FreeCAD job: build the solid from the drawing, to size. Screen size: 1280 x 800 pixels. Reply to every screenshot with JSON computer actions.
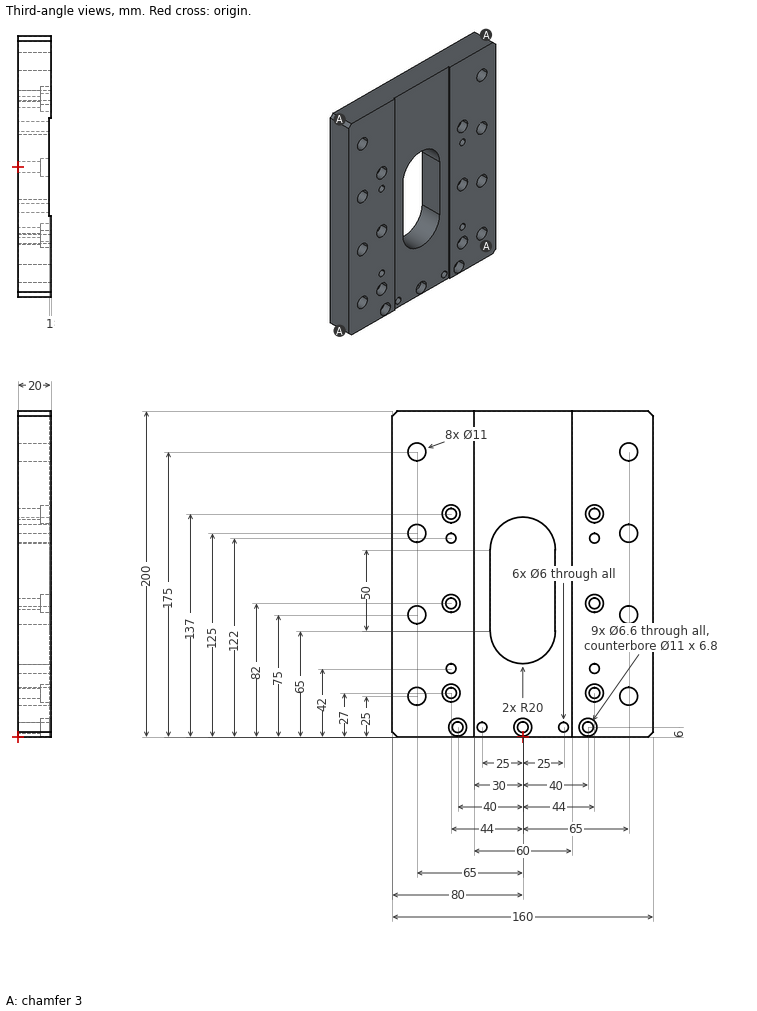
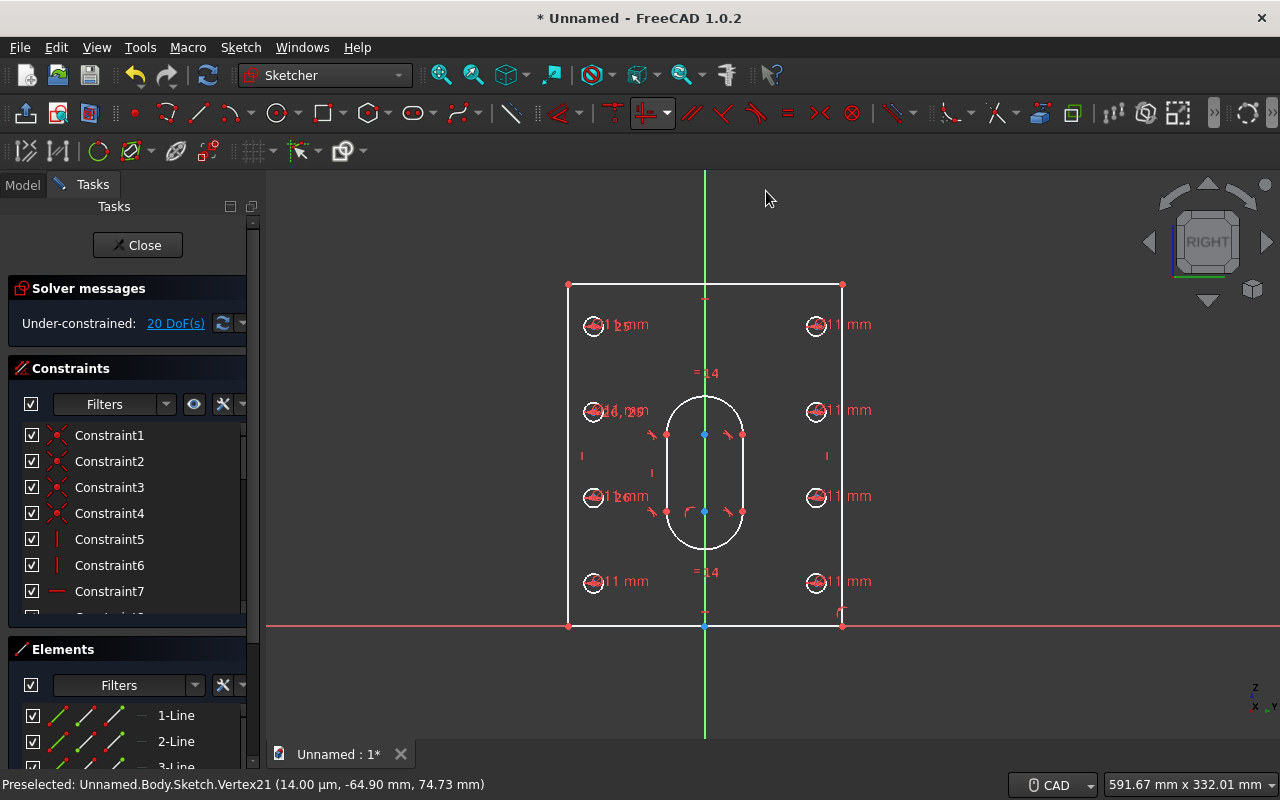
{"action": "left_click", "coordinate": [594, 498]}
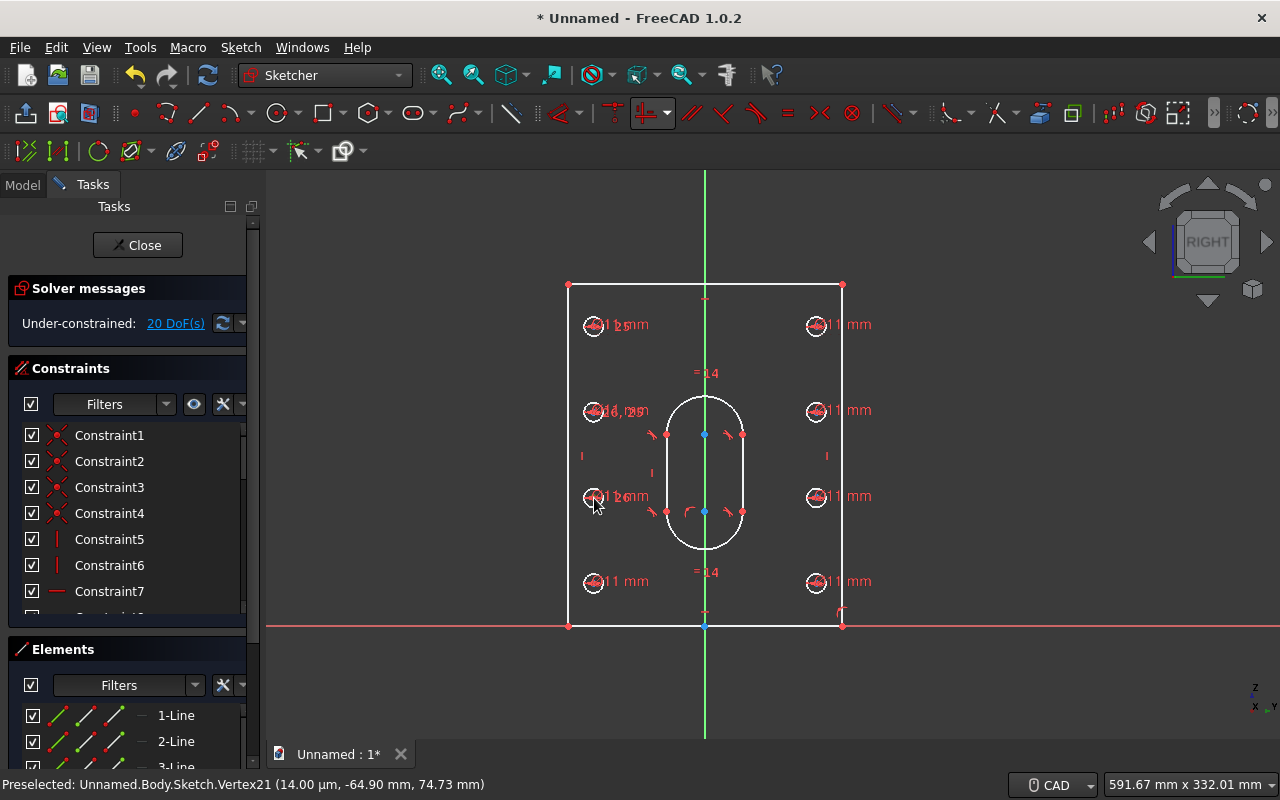
{"action": "left_click", "coordinate": [594, 583]}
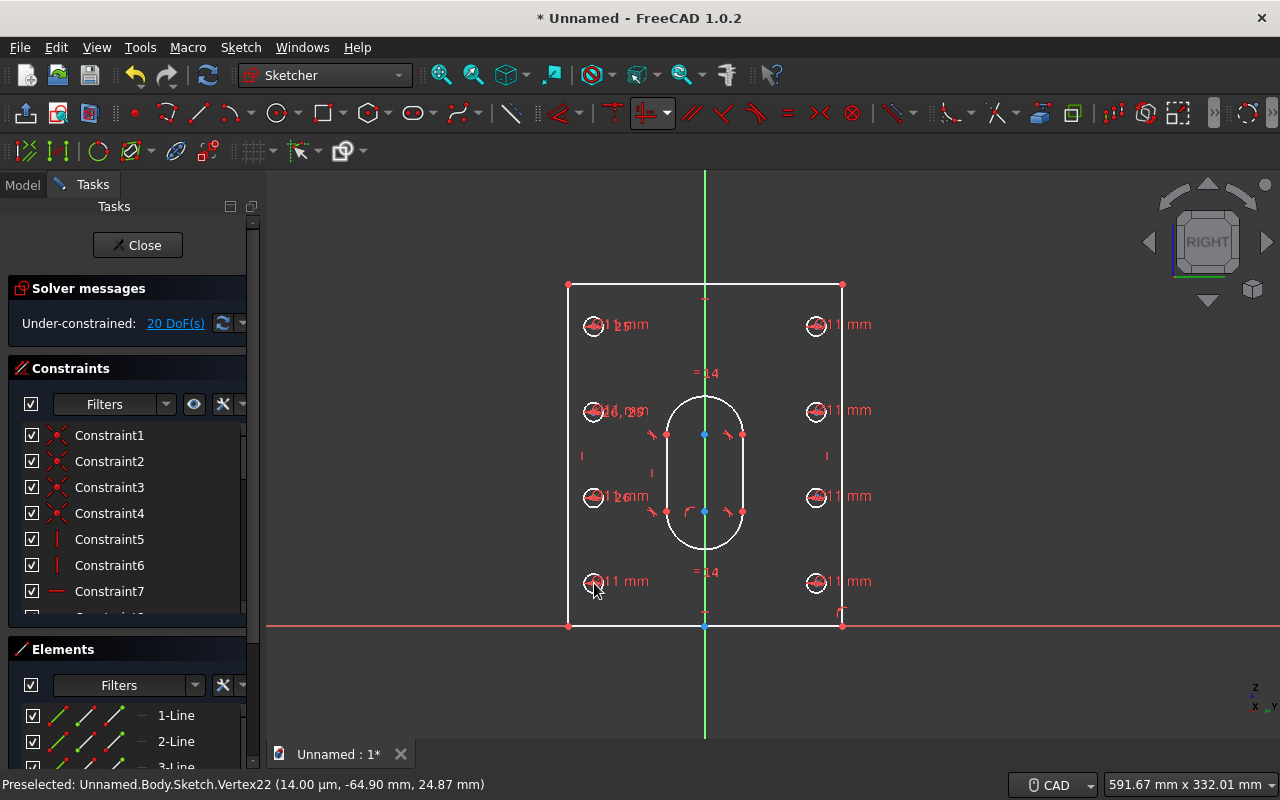
{"action": "key", "text": "v"}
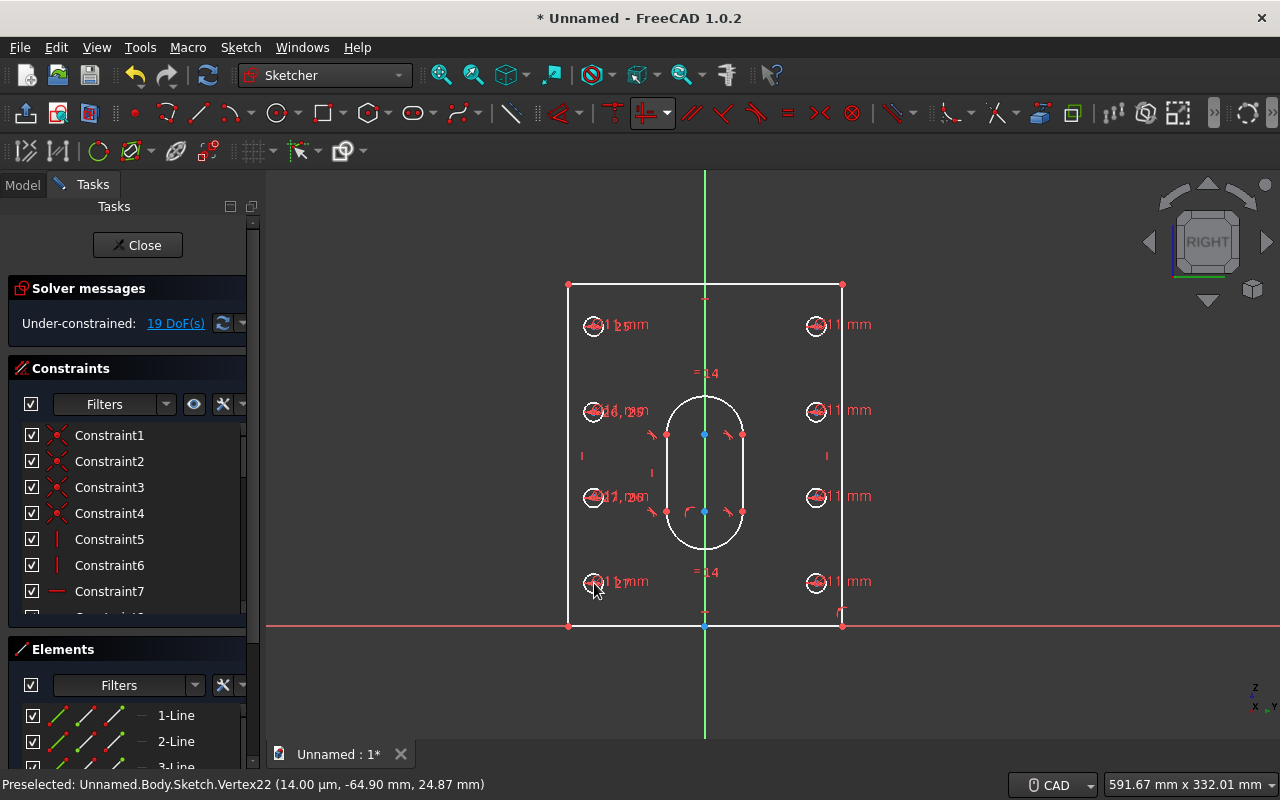
{"action": "left_click", "coordinate": [816, 327]}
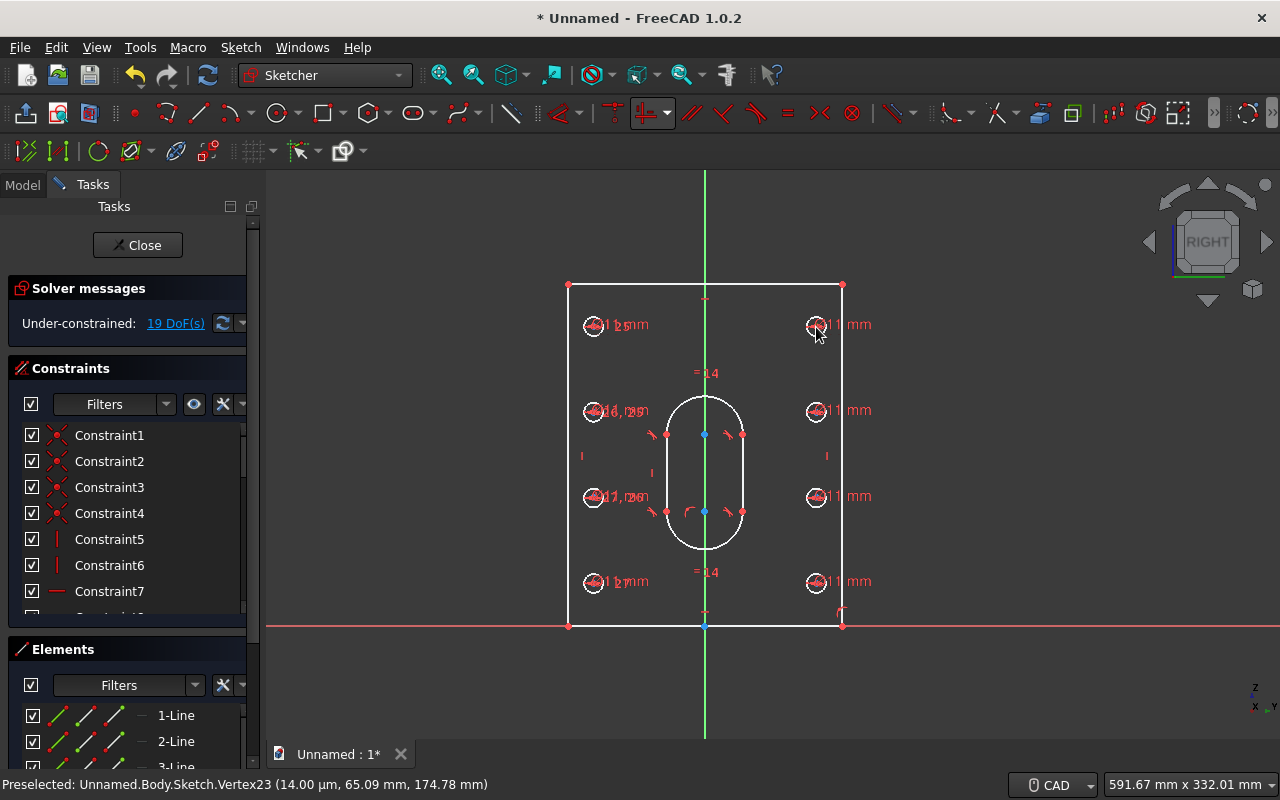
{"action": "left_click", "coordinate": [816, 412]}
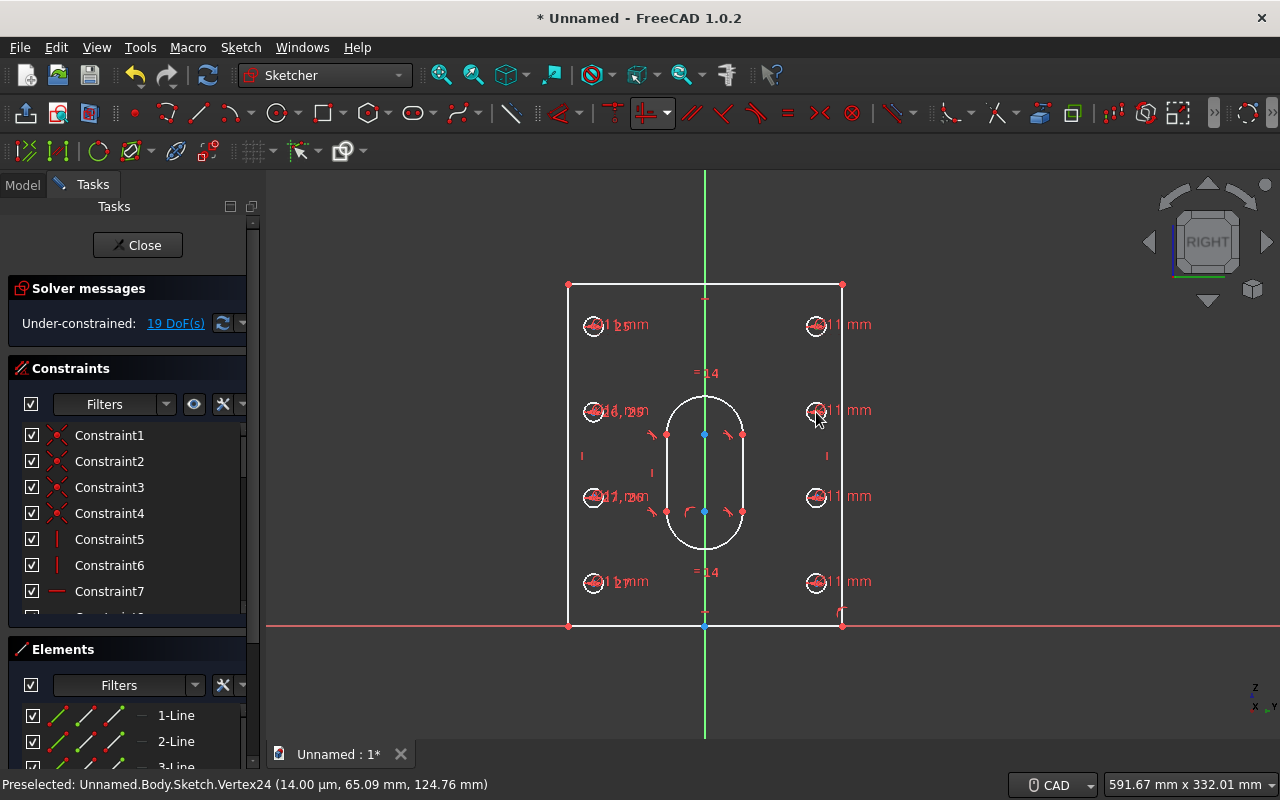
{"action": "key", "text": "v"}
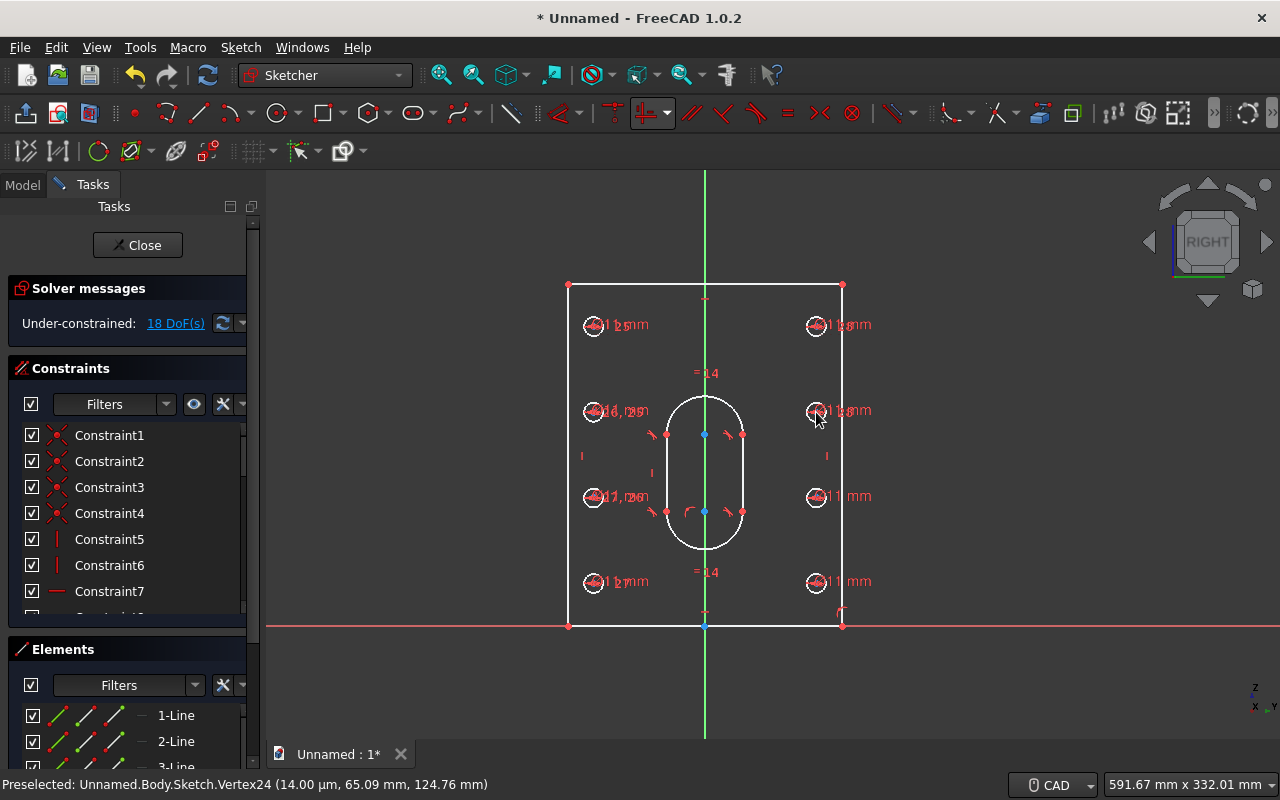
{"action": "left_click", "coordinate": [816, 412]}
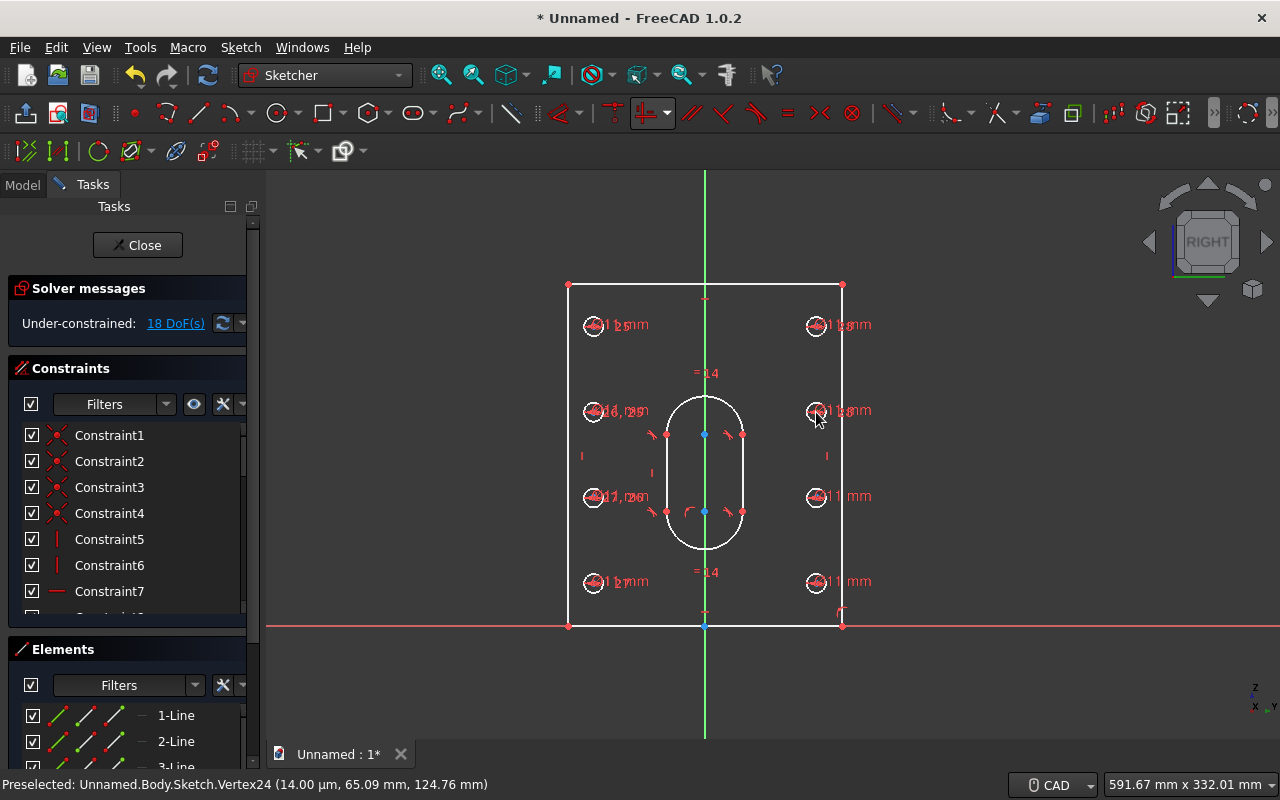
{"action": "left_click", "coordinate": [816, 498]}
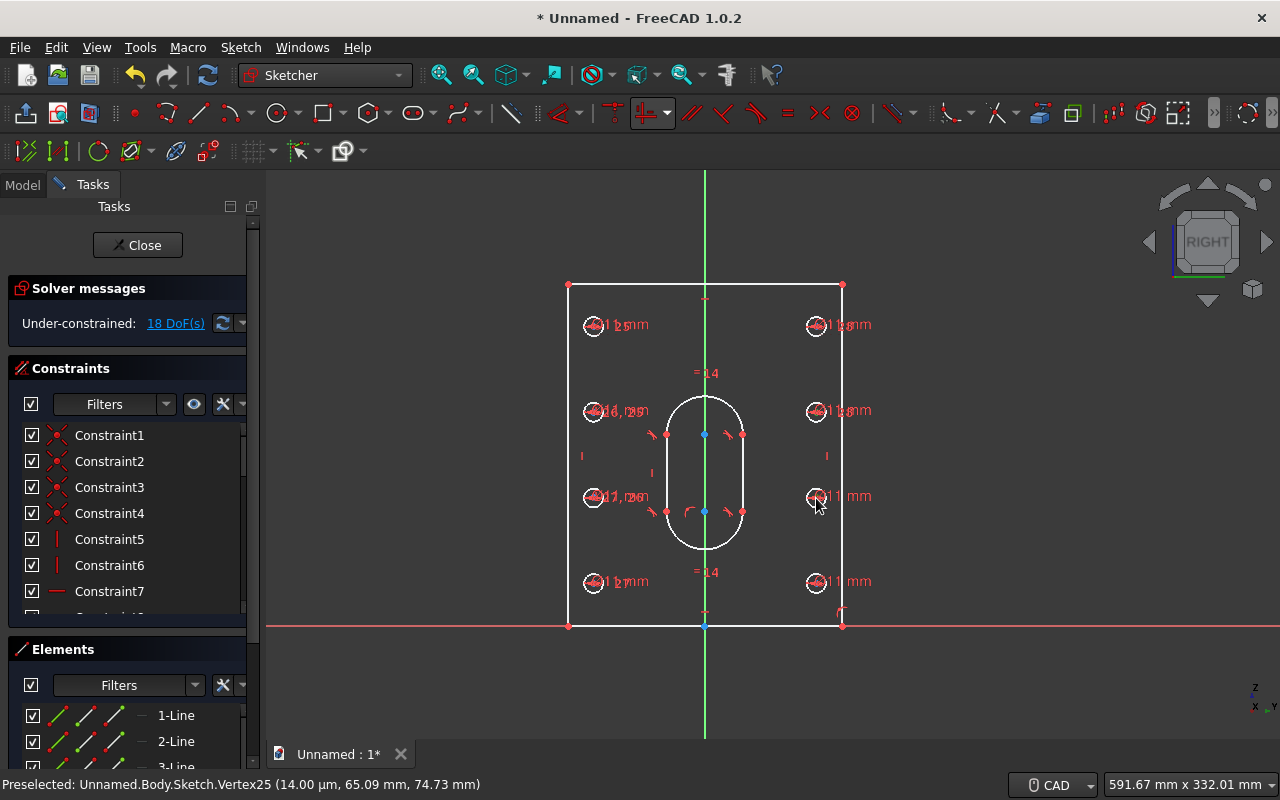
{"action": "key", "text": "v"}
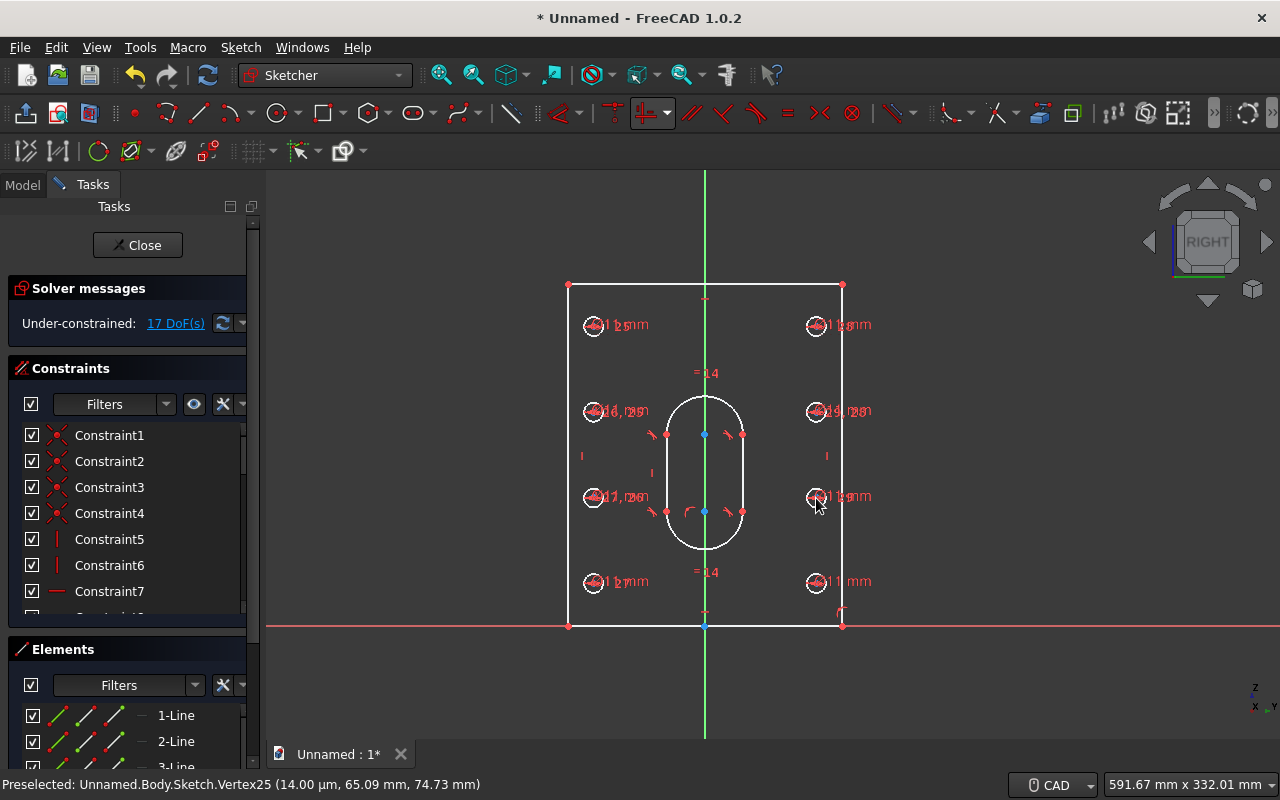
{"action": "left_click", "coordinate": [816, 498]}